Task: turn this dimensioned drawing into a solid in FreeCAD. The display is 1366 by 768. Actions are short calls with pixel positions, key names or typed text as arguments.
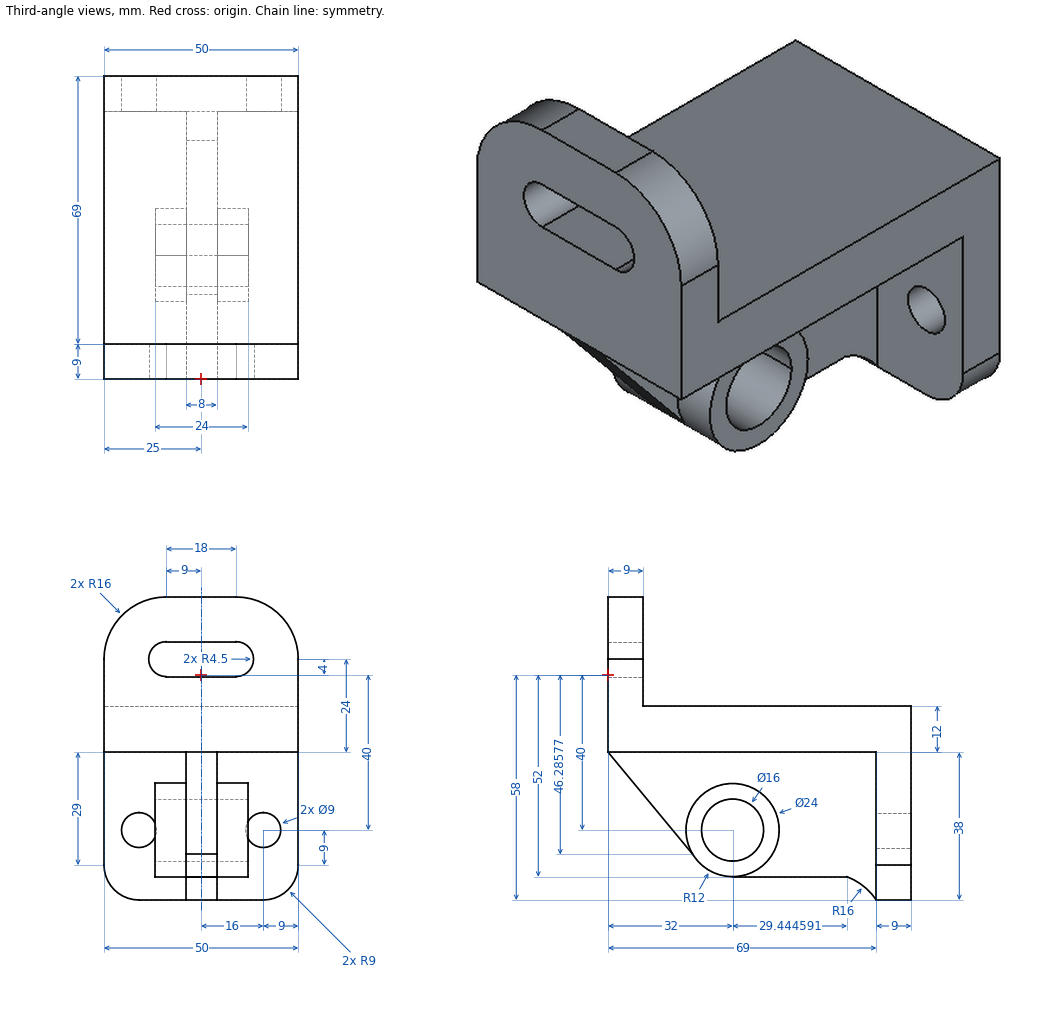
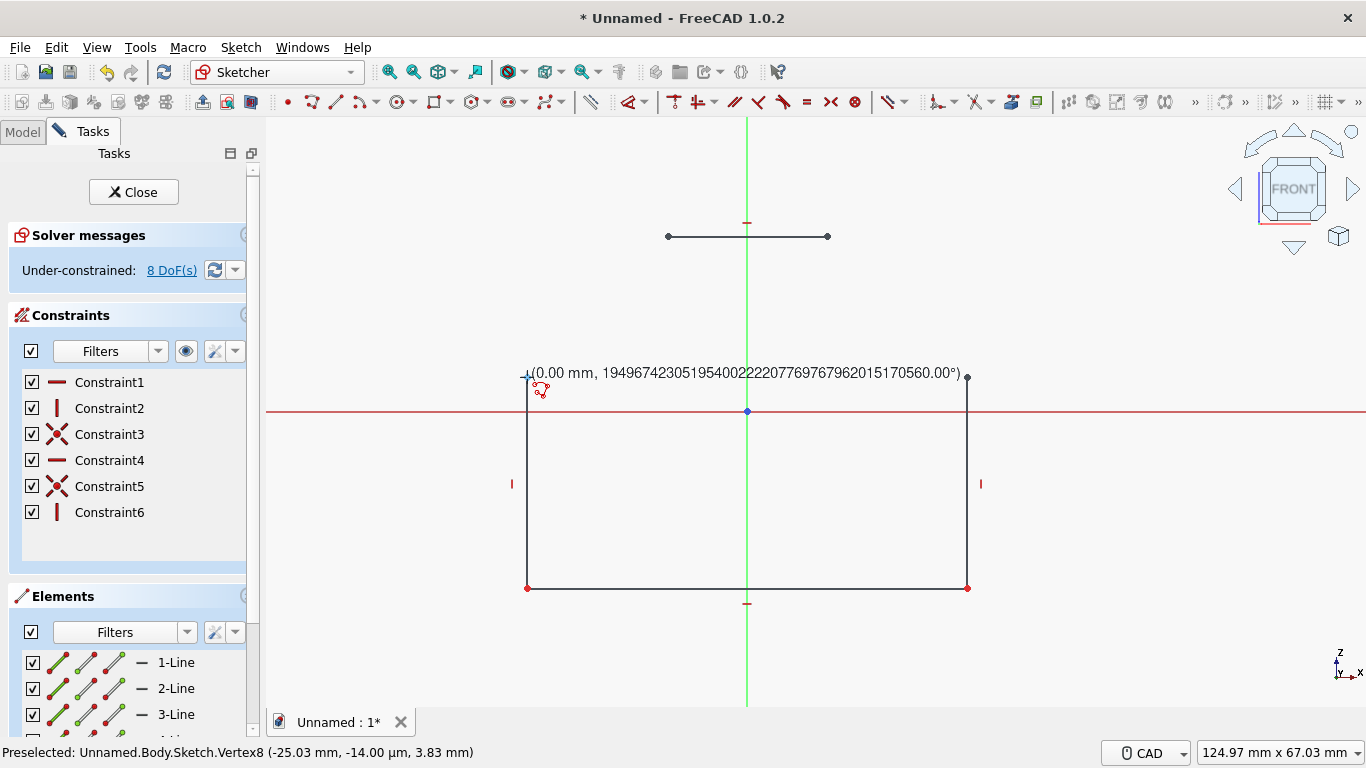
key(g)
key(3)
key(a)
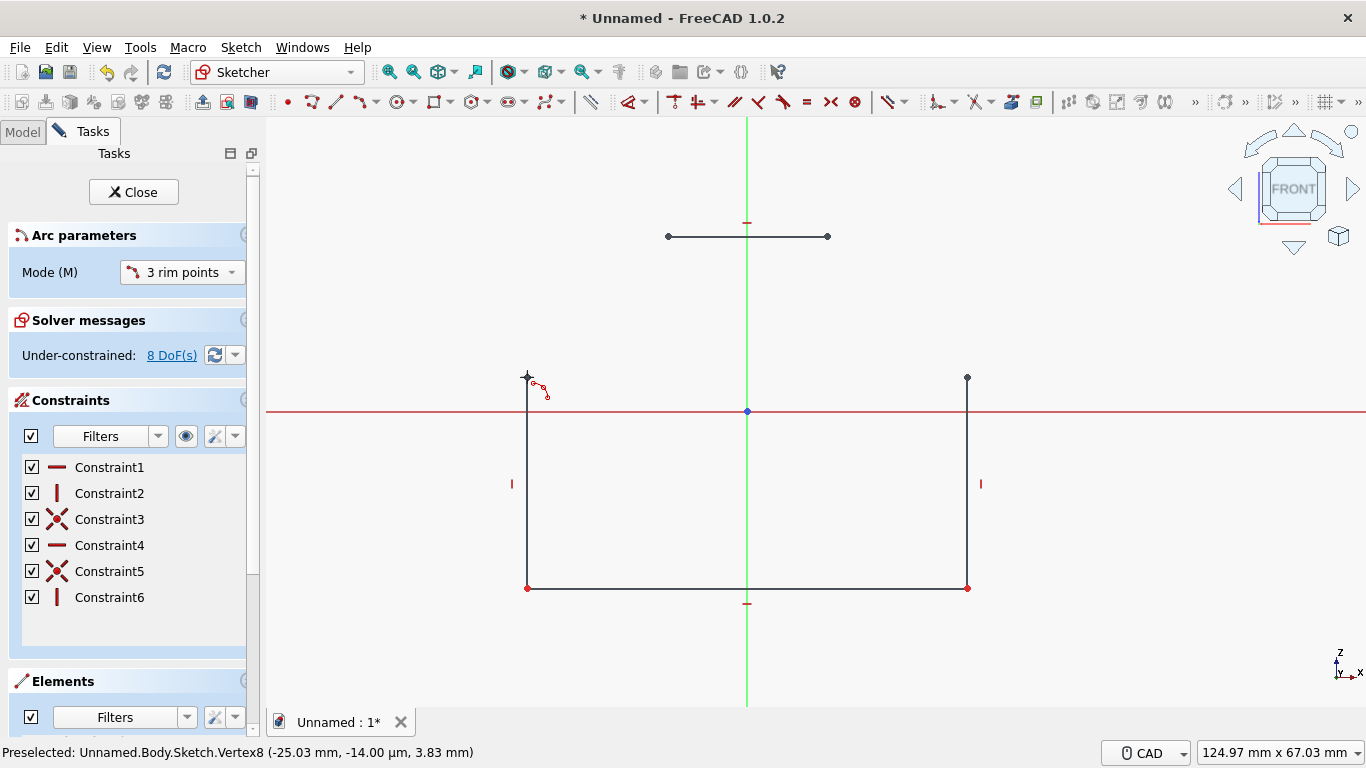
click(827, 237)
click(967, 378)
click(926, 277)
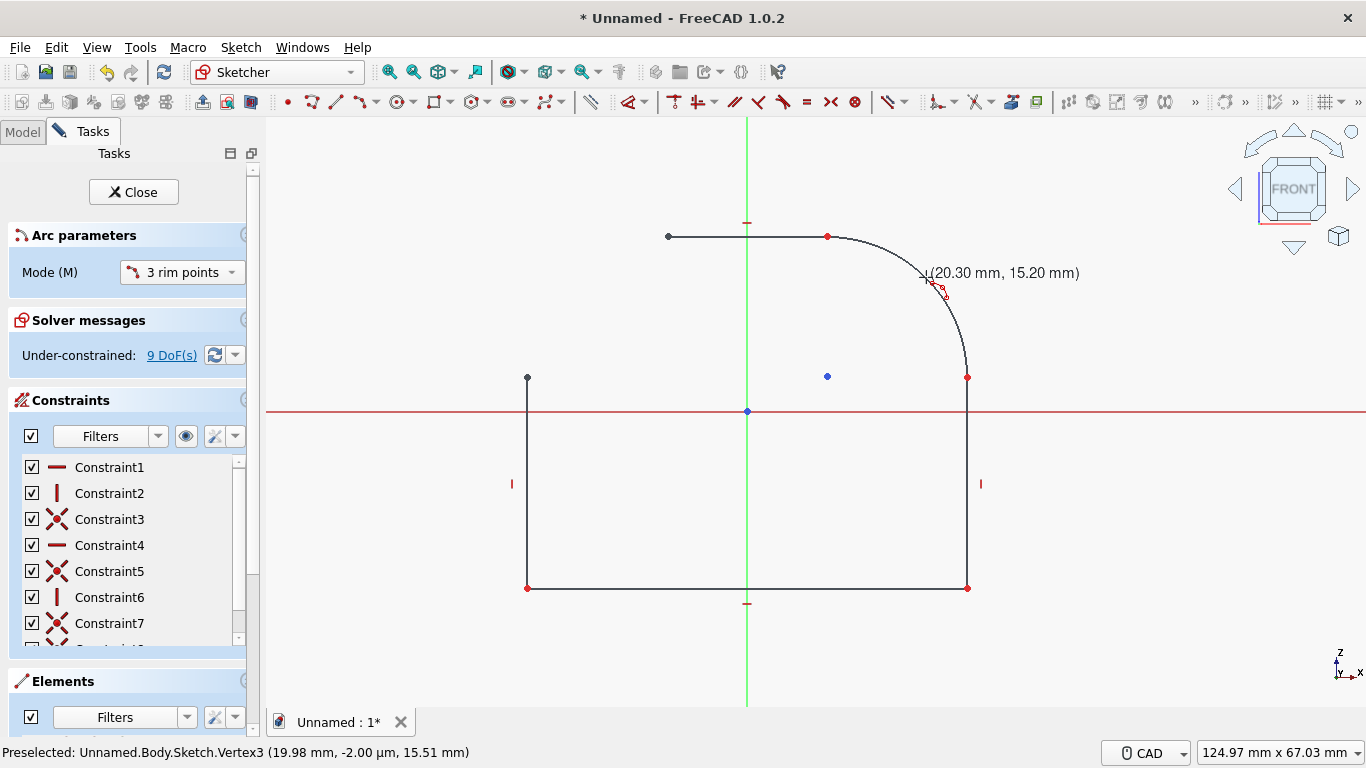
click(527, 378)
click(668, 237)
click(569, 277)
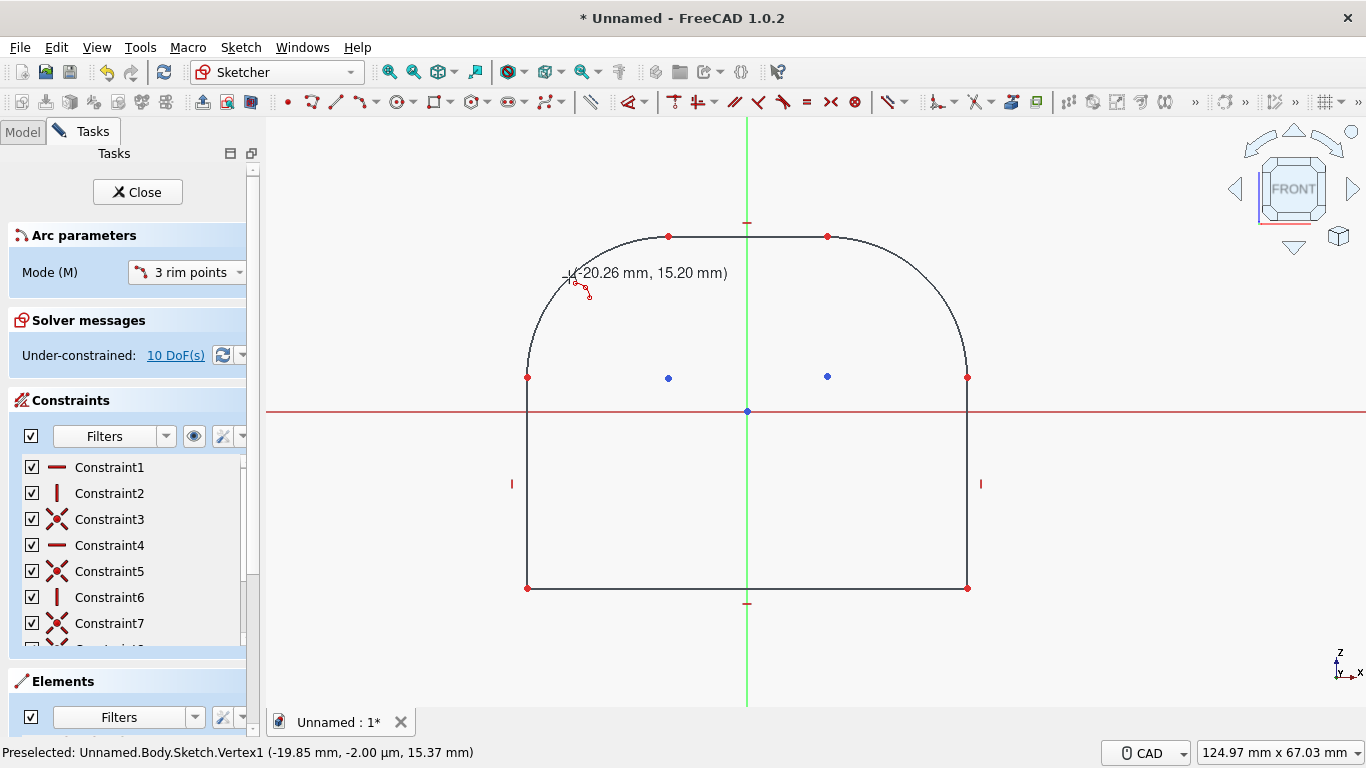
key(g)
key(s)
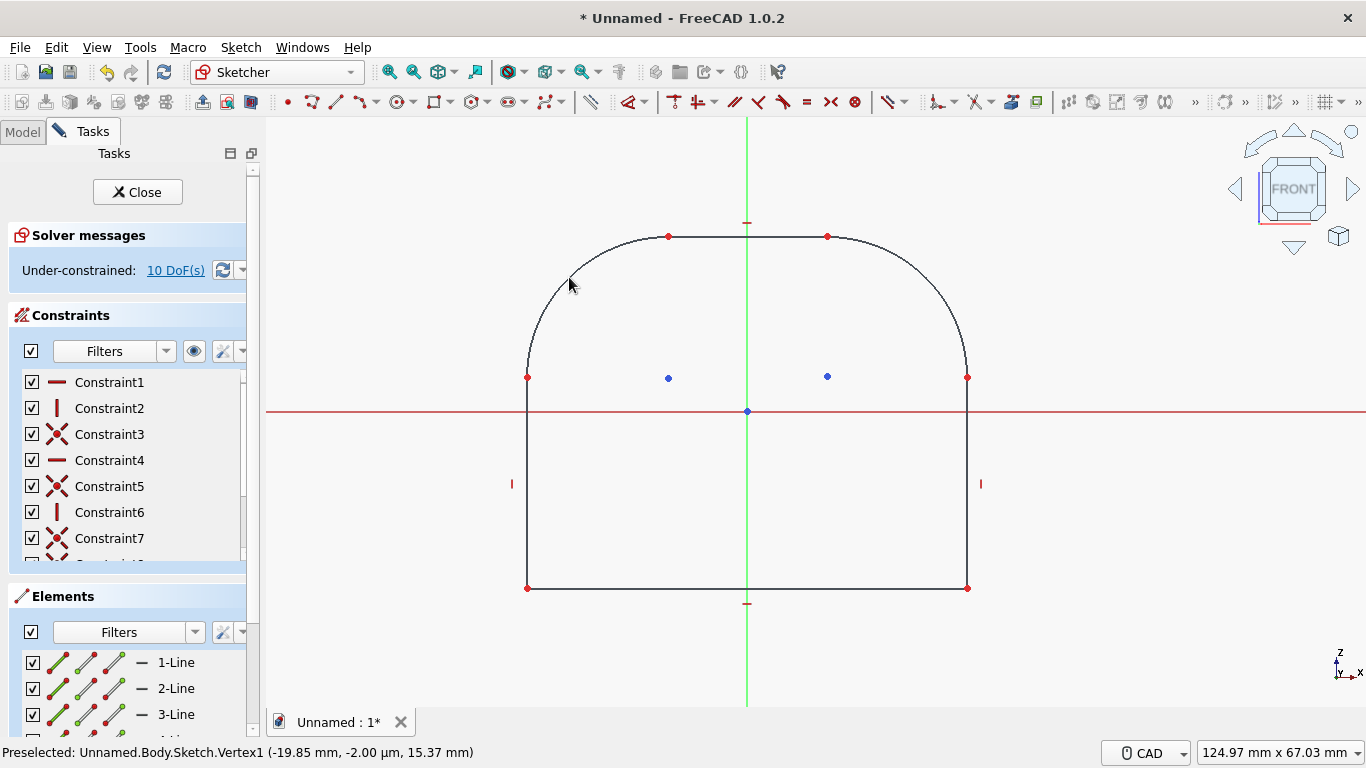
click(668, 377)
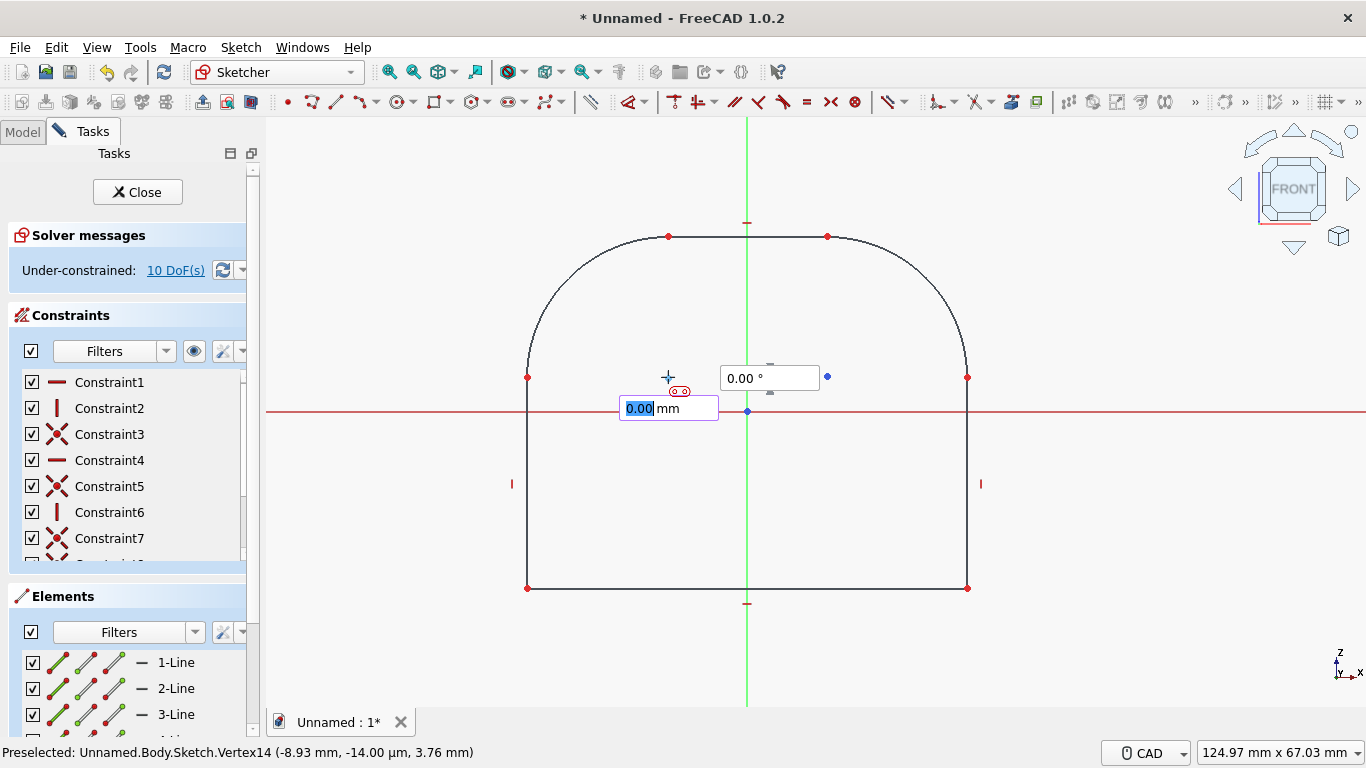
click(827, 377)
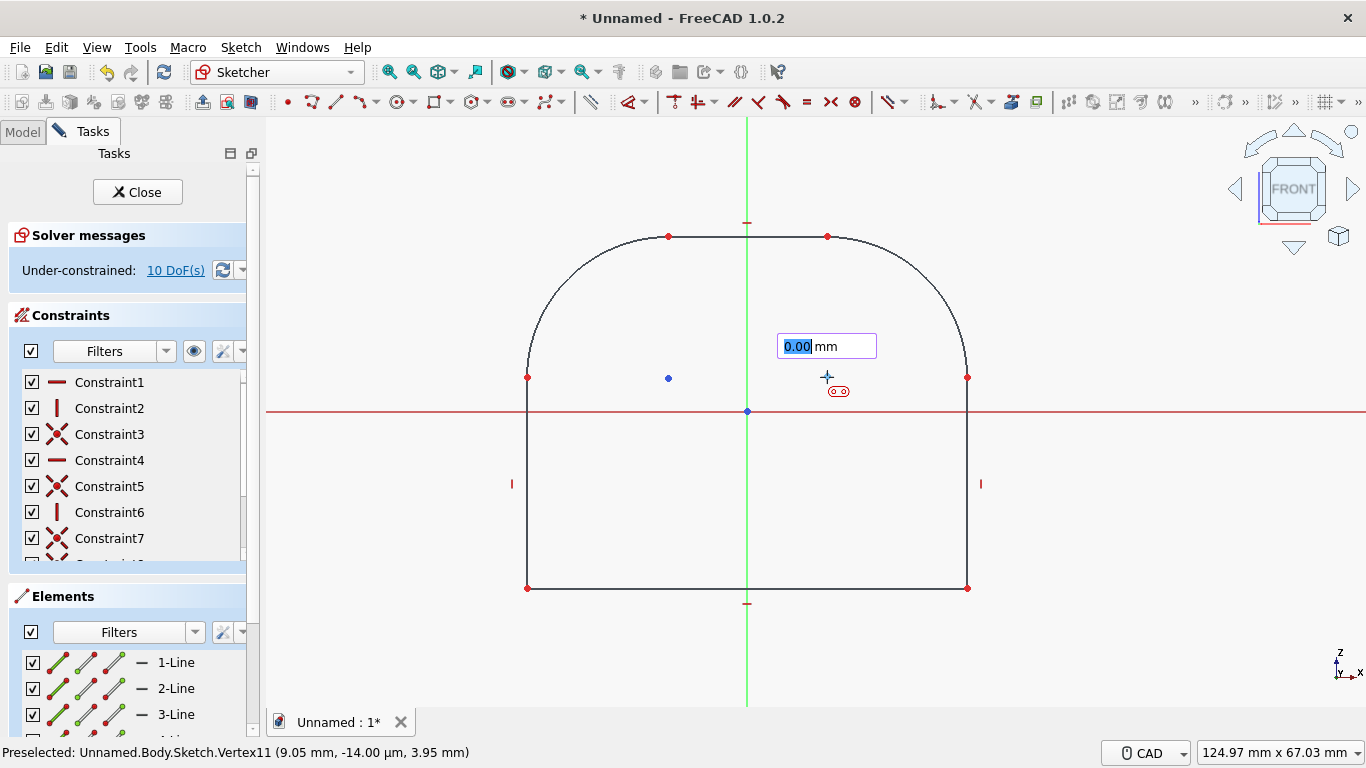
click(771, 337)
key(Escape)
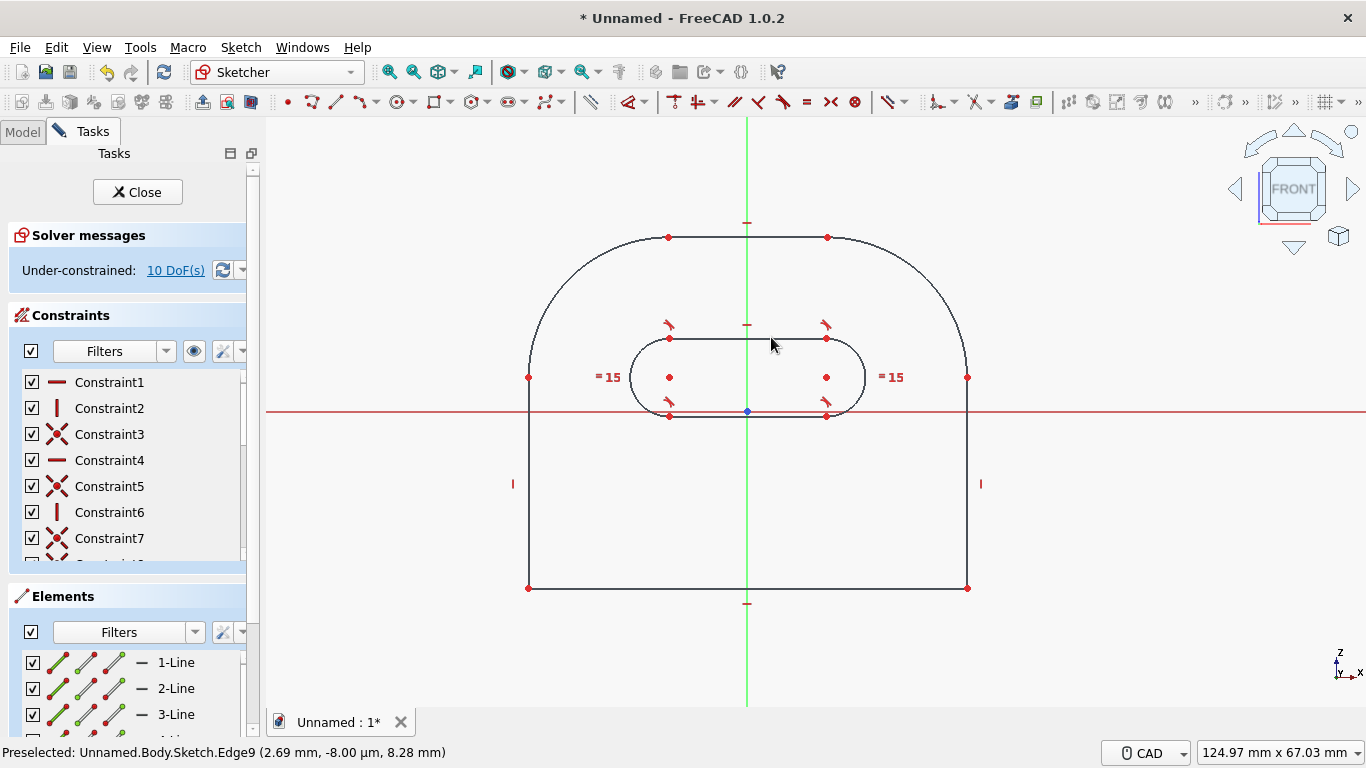
click(716, 237)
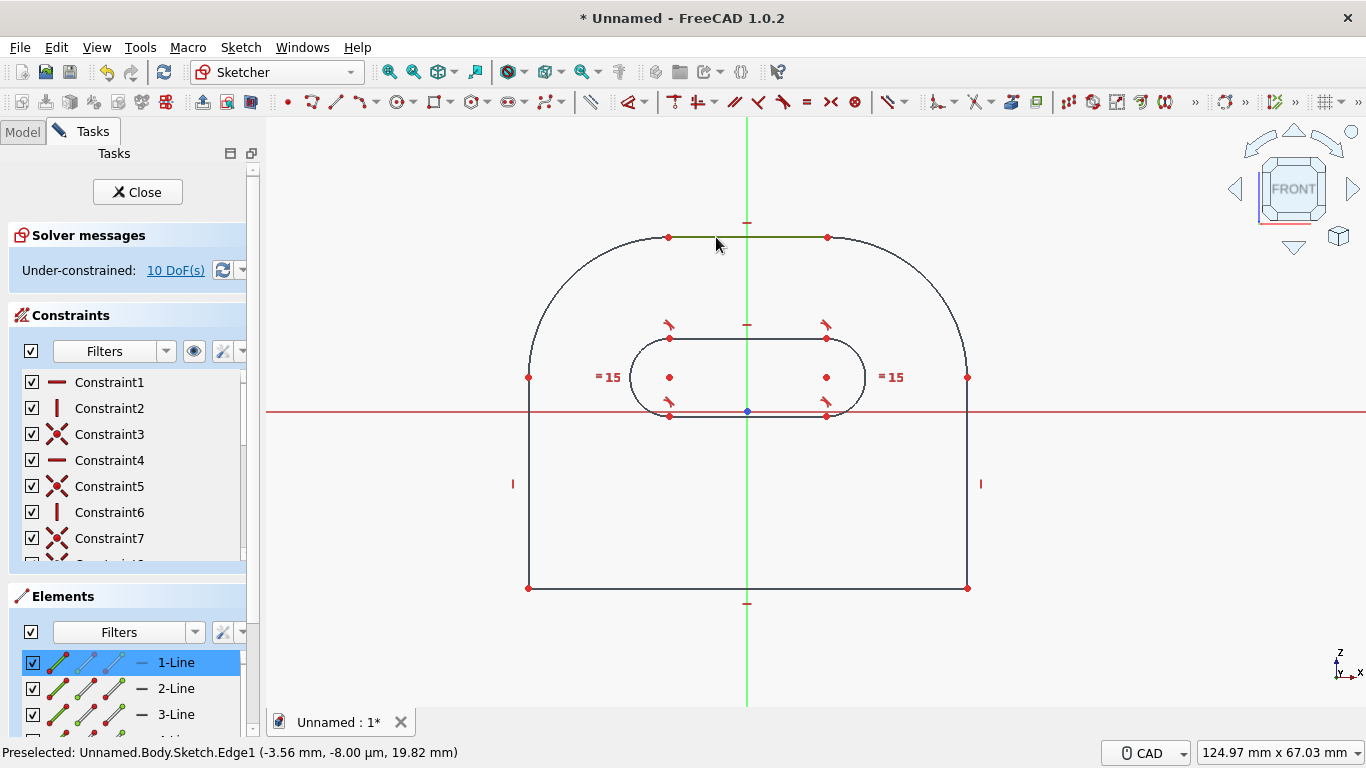
click(952, 314)